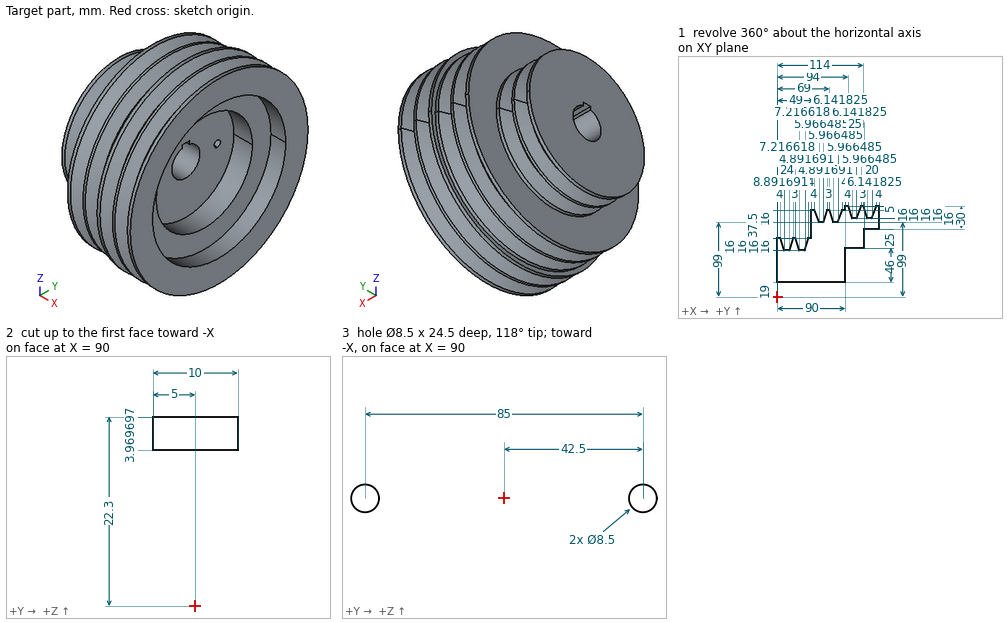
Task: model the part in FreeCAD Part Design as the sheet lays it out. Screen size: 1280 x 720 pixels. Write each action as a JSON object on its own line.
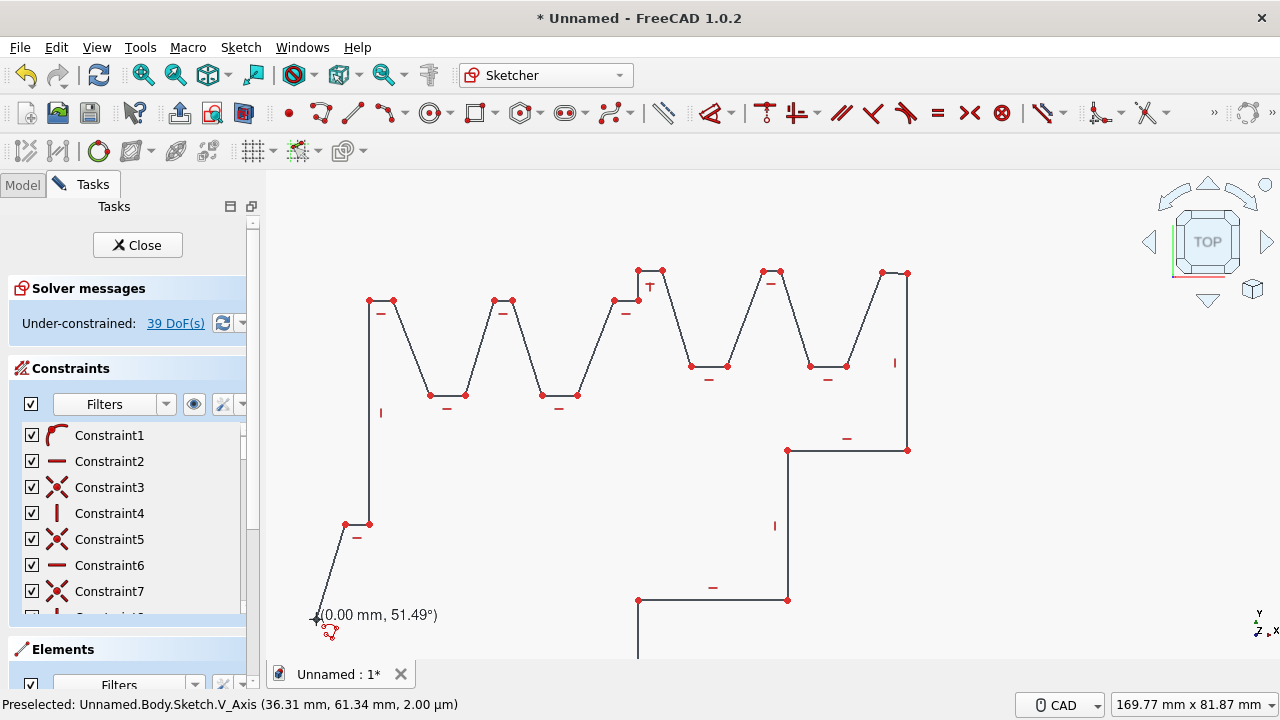
{"action": "scroll", "coordinate": [869, 240], "scroll_direction": "down", "scroll_amount": 4}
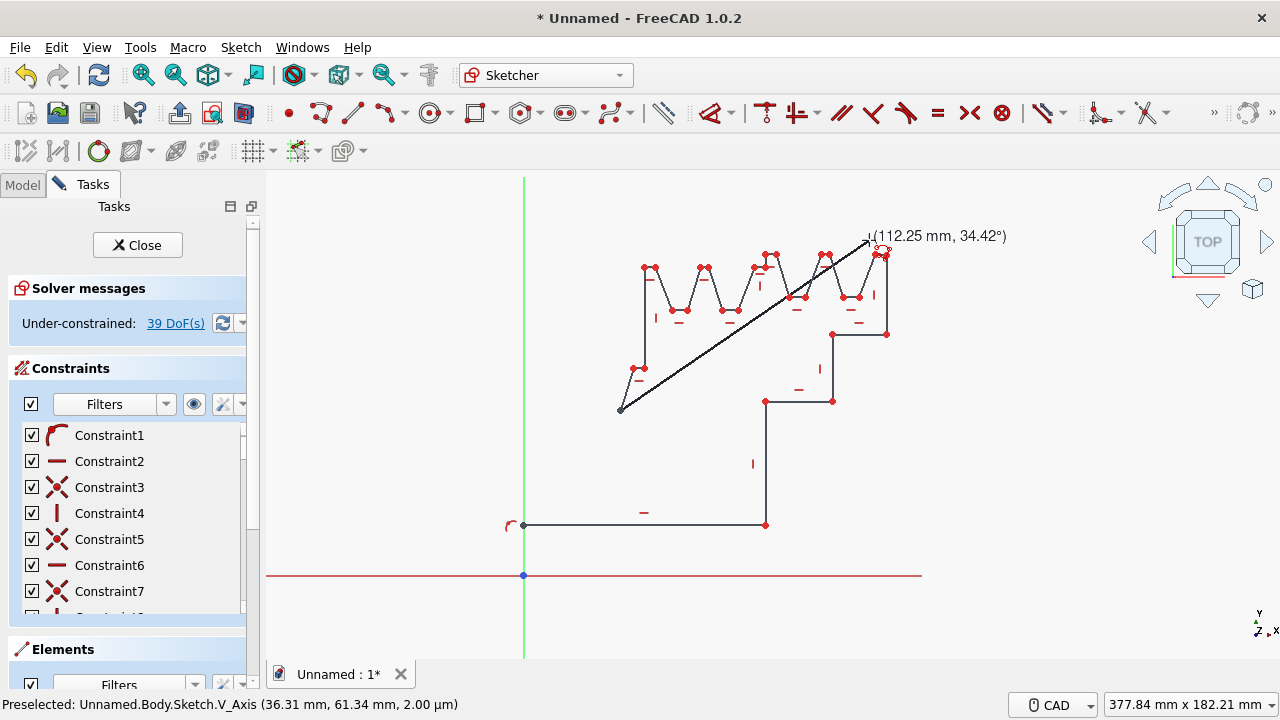
{"action": "left_click", "coordinate": [601, 410]}
{"action": "left_click", "coordinate": [588, 368]}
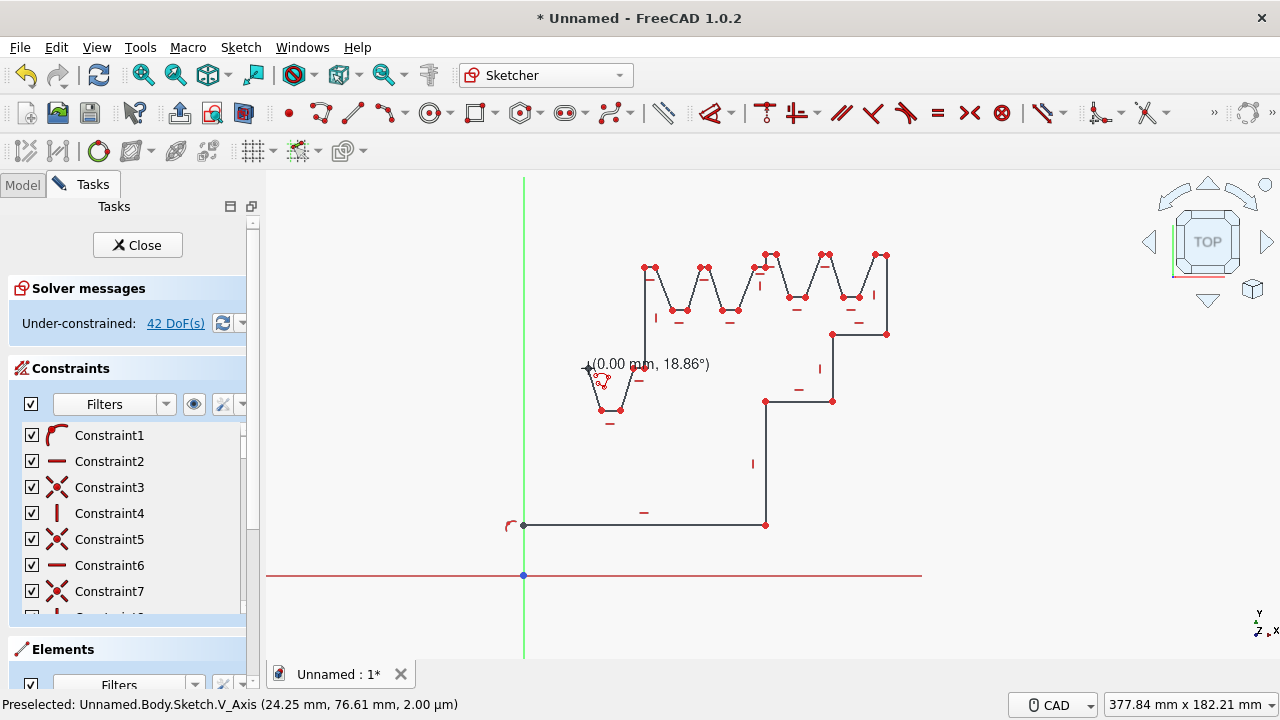
{"action": "scroll", "coordinate": [580, 368], "scroll_direction": "up", "scroll_amount": 4}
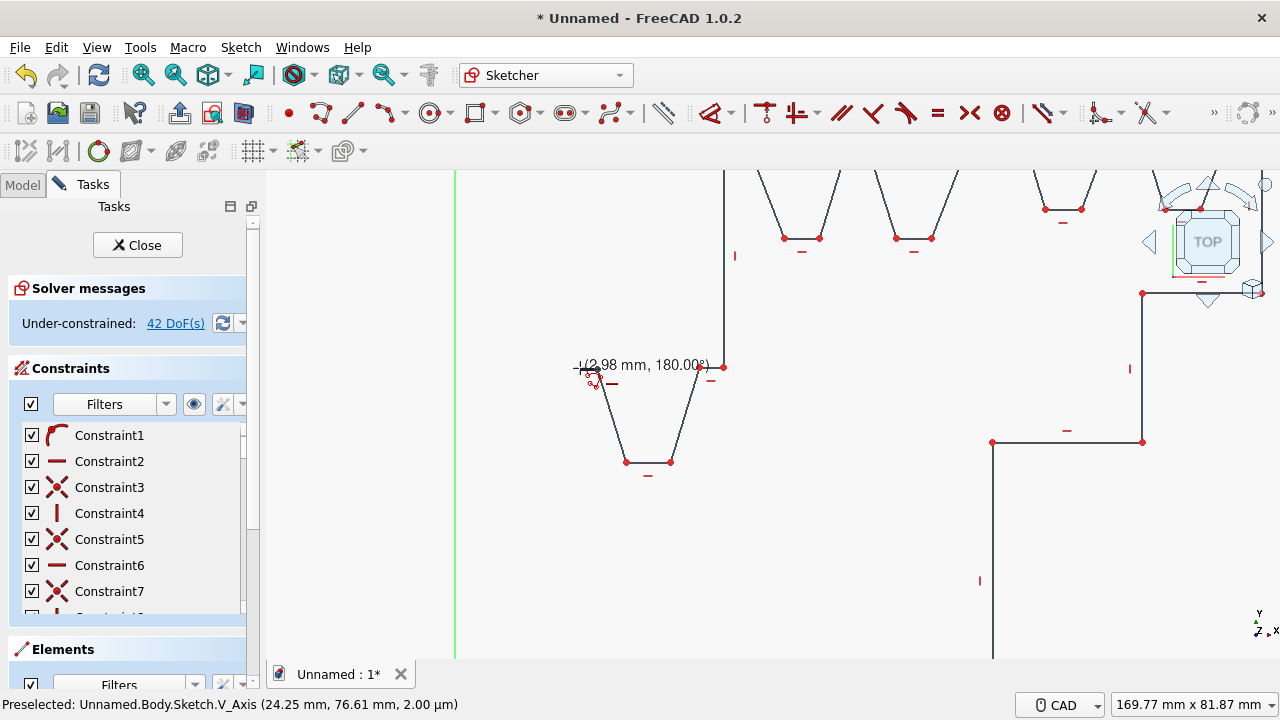
{"action": "left_click", "coordinate": [580, 368]}
{"action": "left_click", "coordinate": [551, 462]}
{"action": "left_click", "coordinate": [508, 462]}
{"action": "left_click", "coordinate": [479, 367]}
{"action": "left_click", "coordinate": [464, 367]}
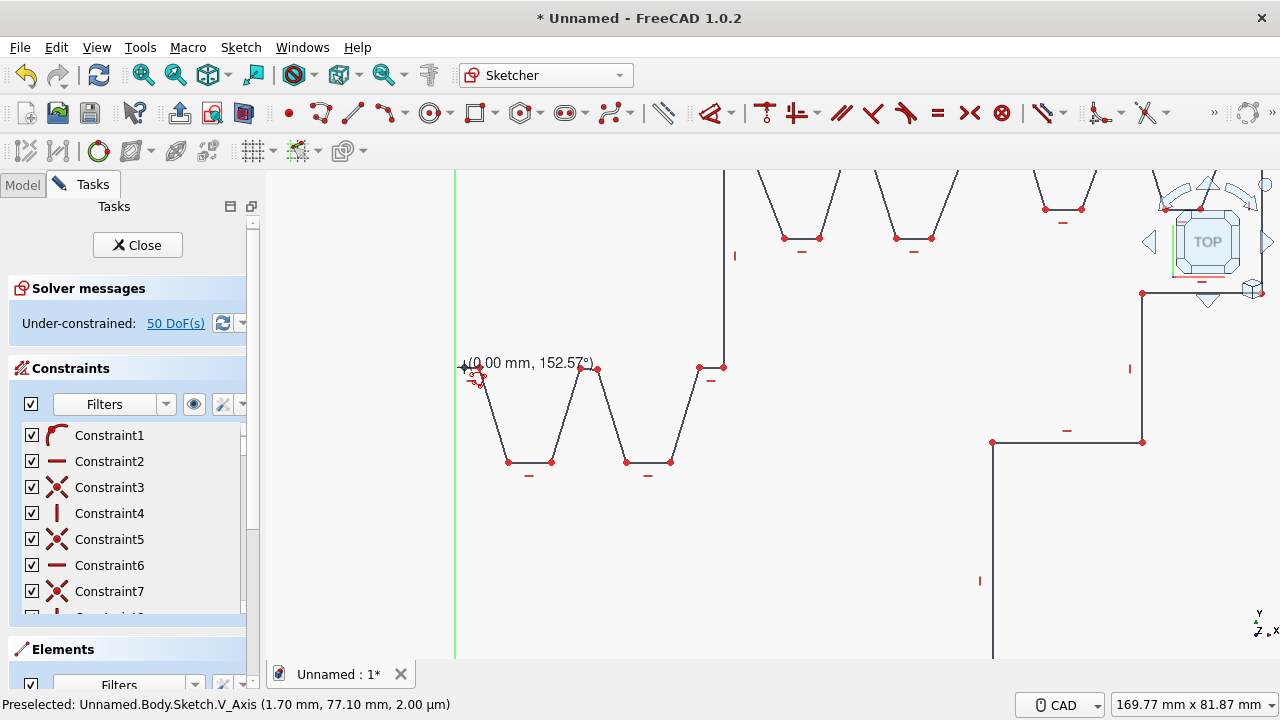
{"action": "scroll", "coordinate": [579, 368], "scroll_direction": "down", "scroll_amount": 4}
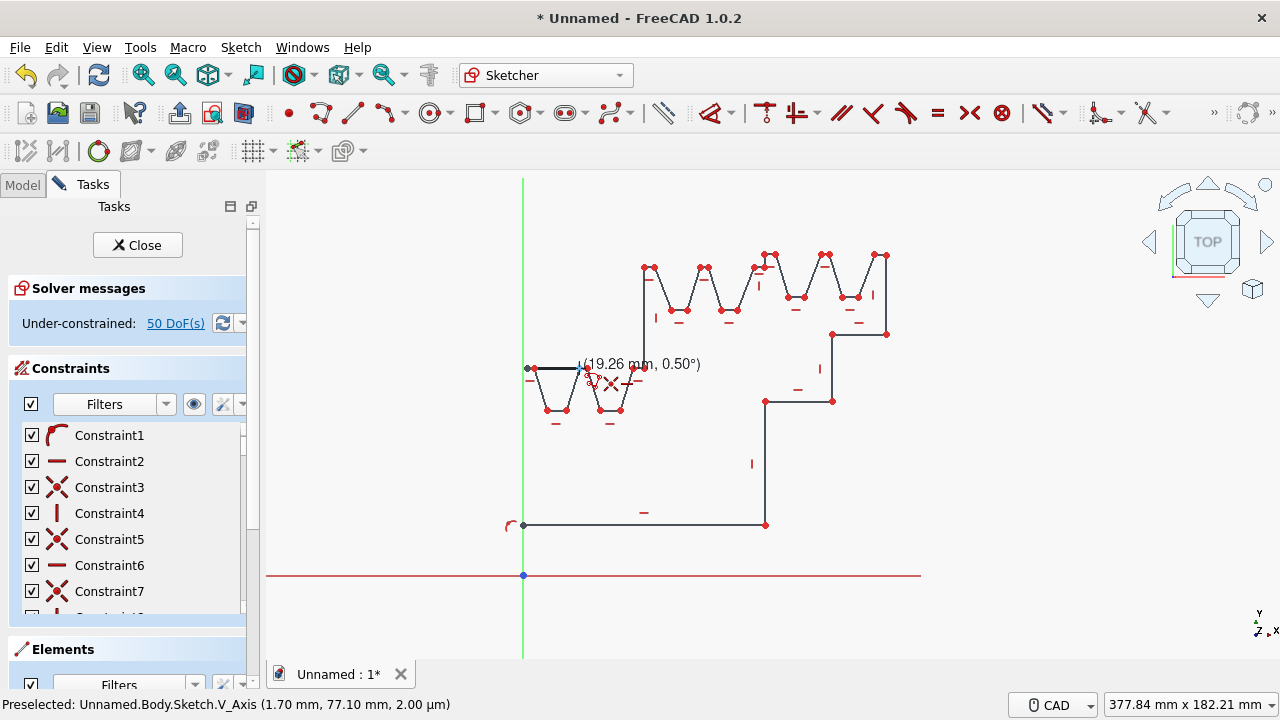
{"action": "left_click", "coordinate": [523, 525]}
{"action": "key", "text": "Escape"}
{"action": "key", "text": "Escape"}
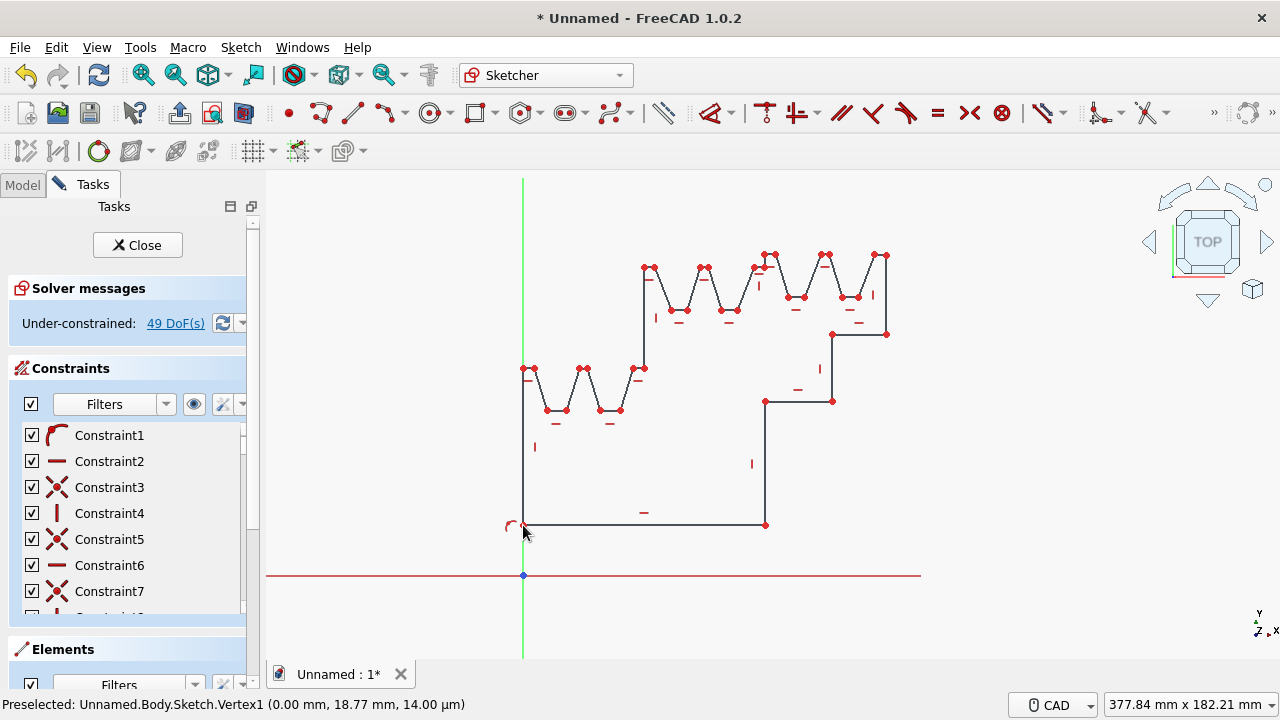
{"action": "scroll", "coordinate": [880, 255], "scroll_direction": "up", "scroll_amount": 5}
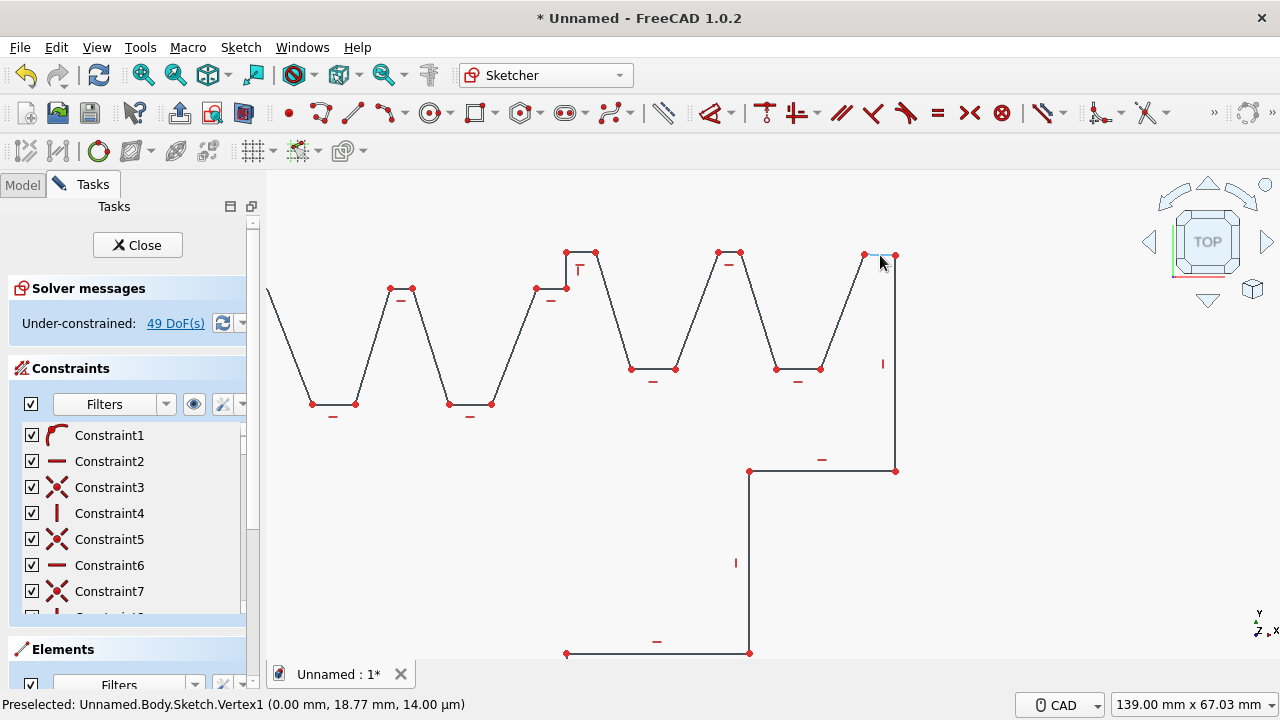
{"action": "left_click", "coordinate": [880, 255]}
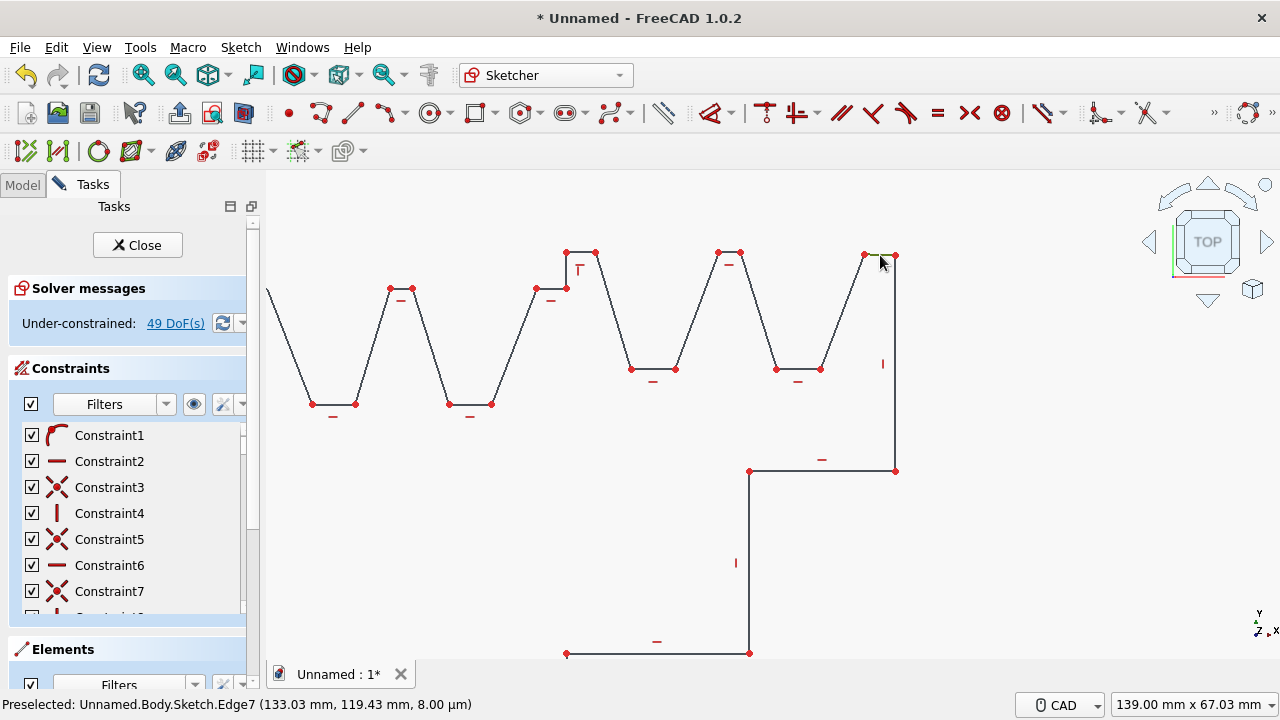
{"action": "key", "text": "h"}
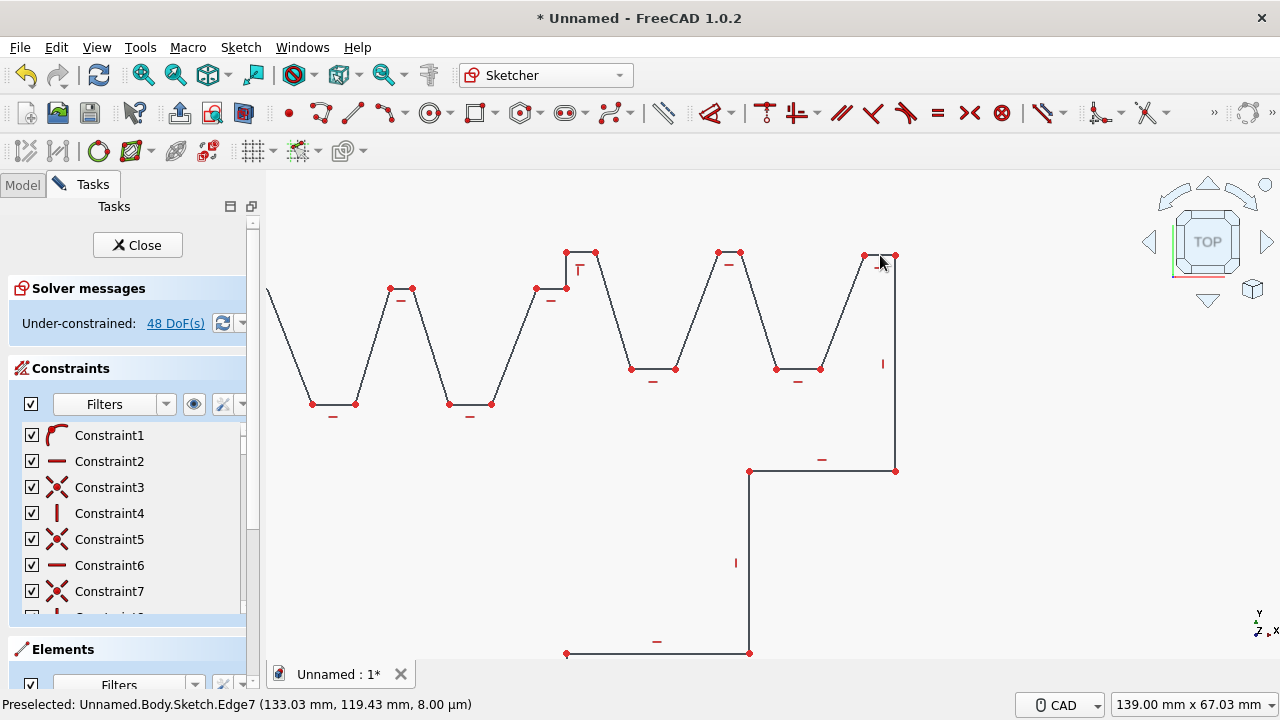
{"action": "scroll", "coordinate": [881, 255], "scroll_direction": "down", "scroll_amount": 5}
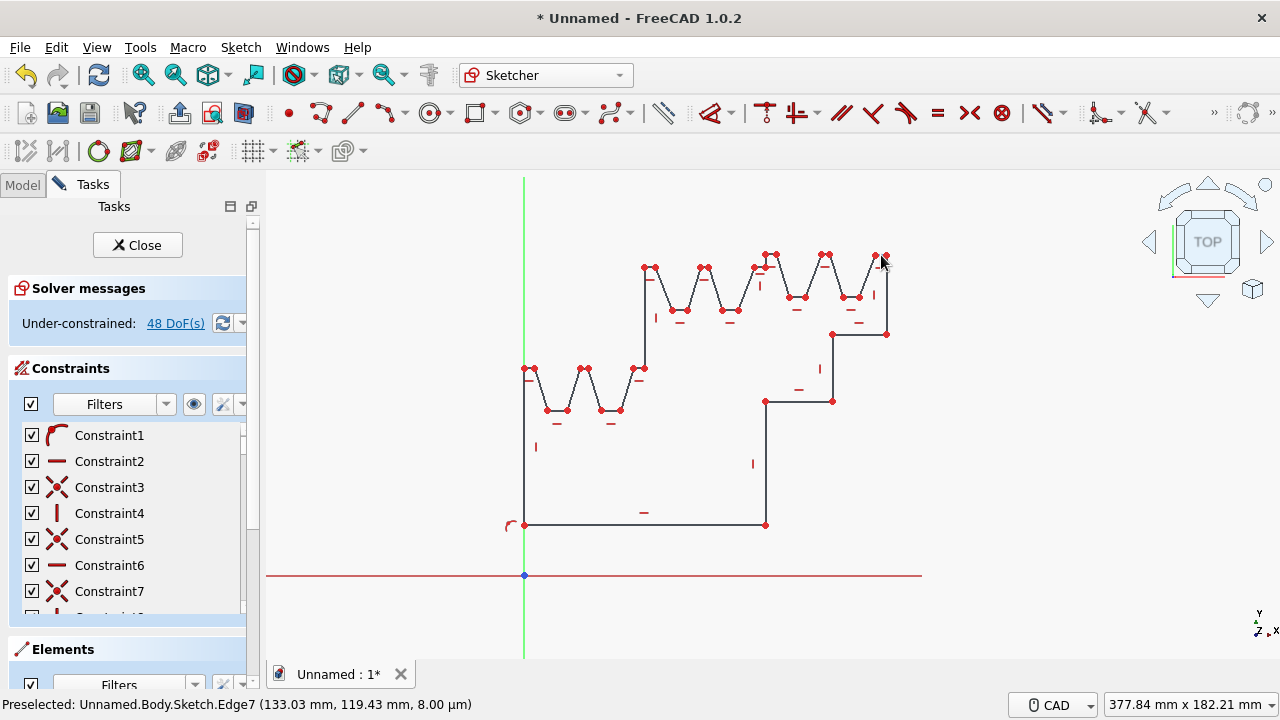
{"action": "scroll", "coordinate": [584, 369], "scroll_direction": "up", "scroll_amount": 7}